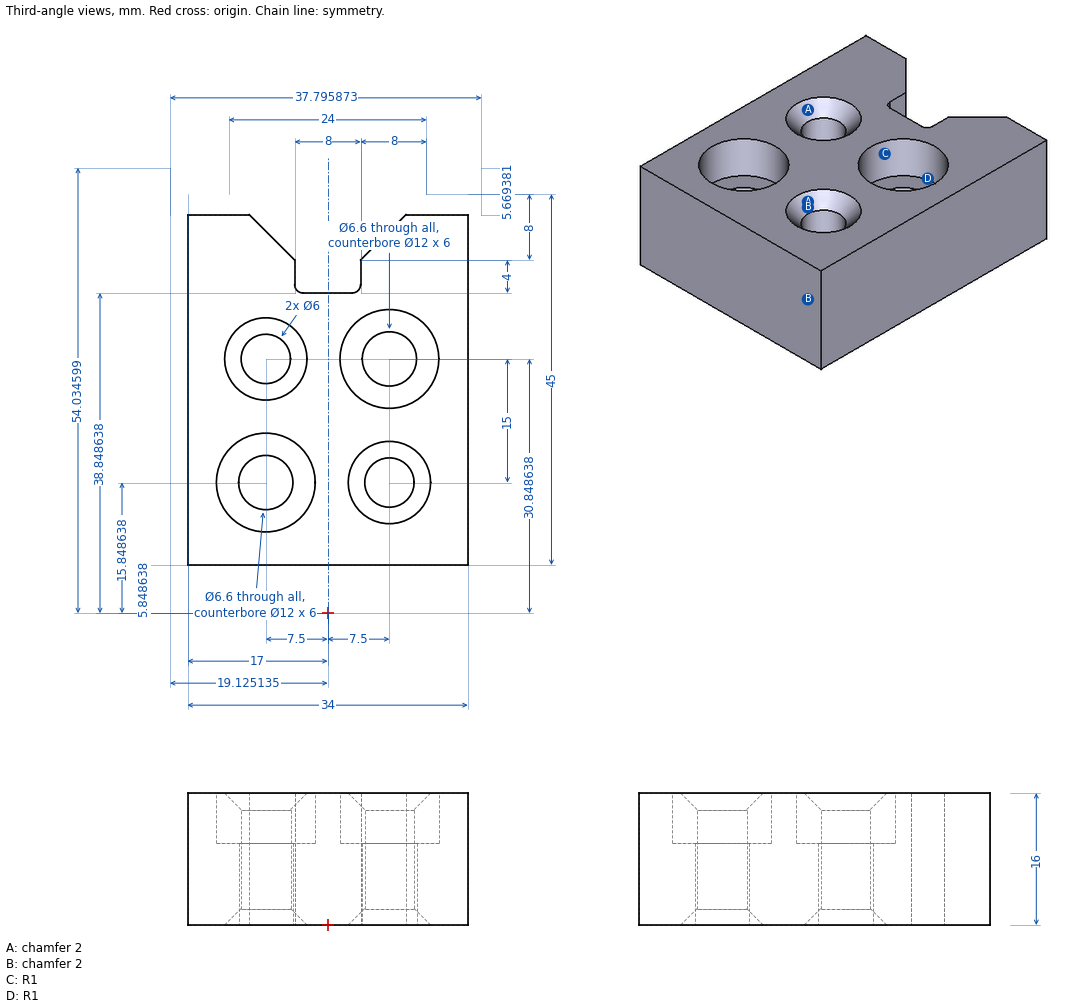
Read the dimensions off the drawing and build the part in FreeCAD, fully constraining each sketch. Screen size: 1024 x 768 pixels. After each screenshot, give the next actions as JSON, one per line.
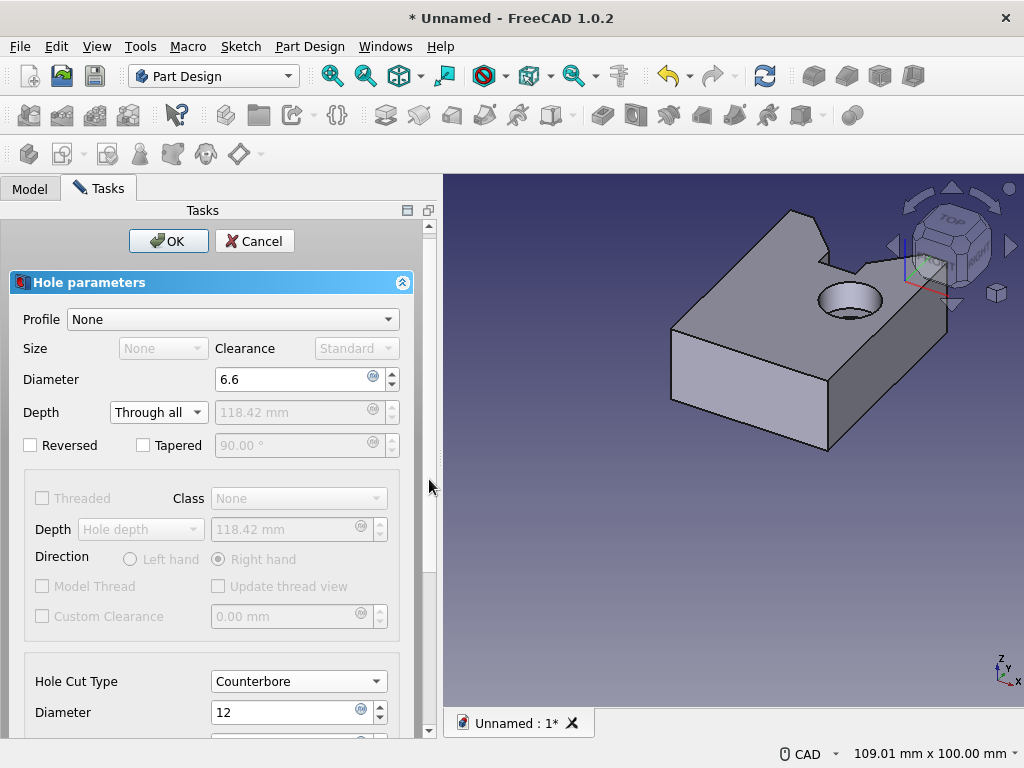
{"action": "left_click", "coordinate": [169, 249]}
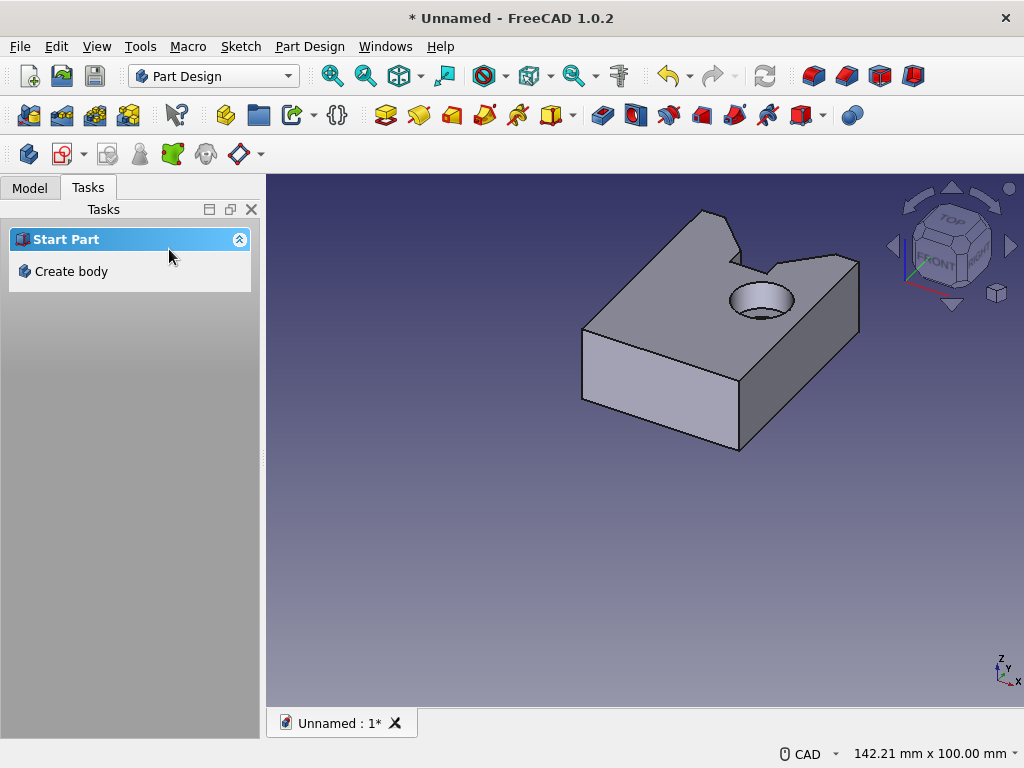
{"action": "left_click", "coordinate": [686, 329]}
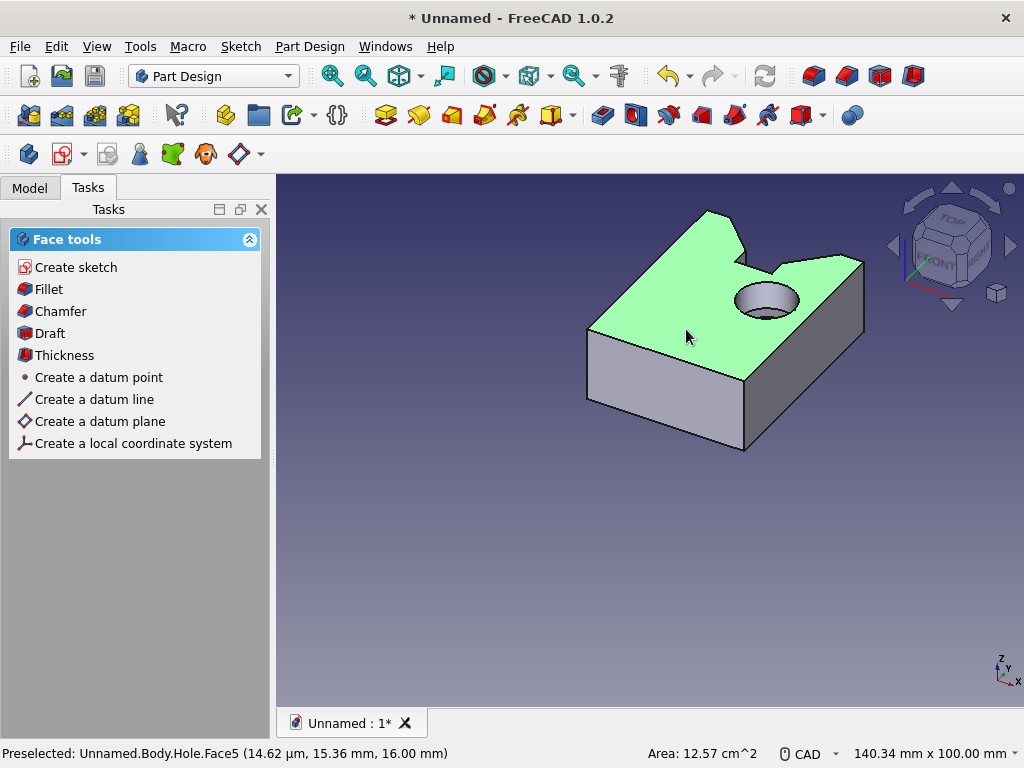
{"action": "left_click", "coordinate": [62, 154]}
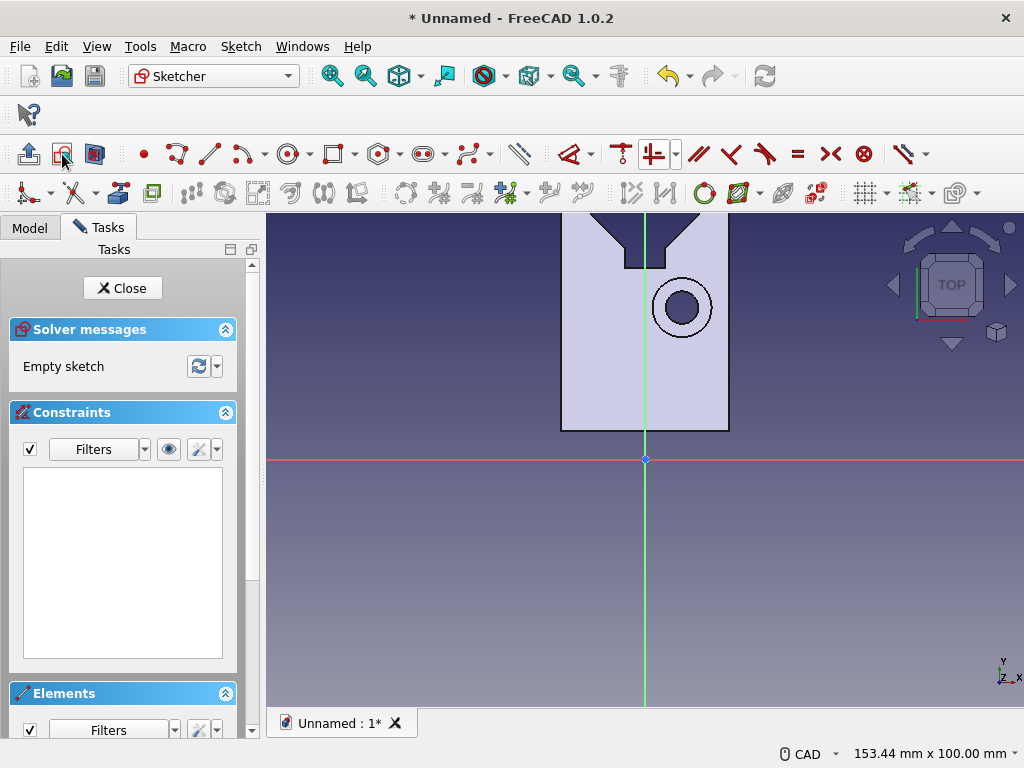
{"action": "scroll", "coordinate": [728, 275], "scroll_direction": "up", "scroll_amount": 3}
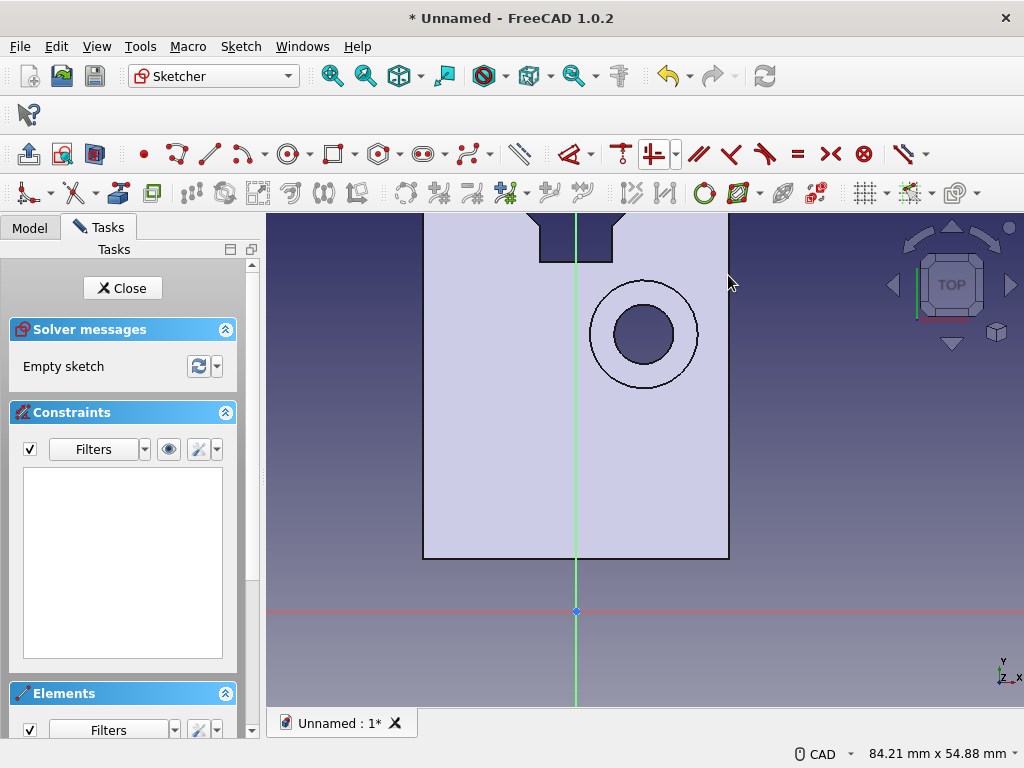
{"action": "left_click", "coordinate": [288, 154]}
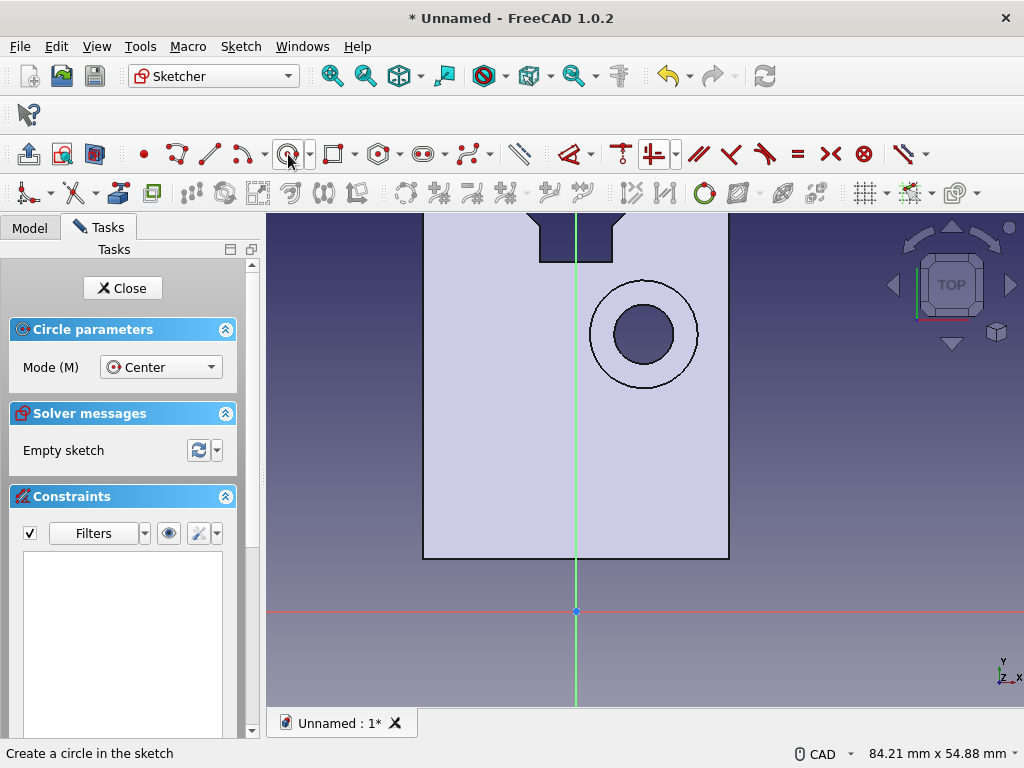
{"action": "left_click", "coordinate": [509, 334]}
{"action": "mouse_move", "coordinate": [528, 315]}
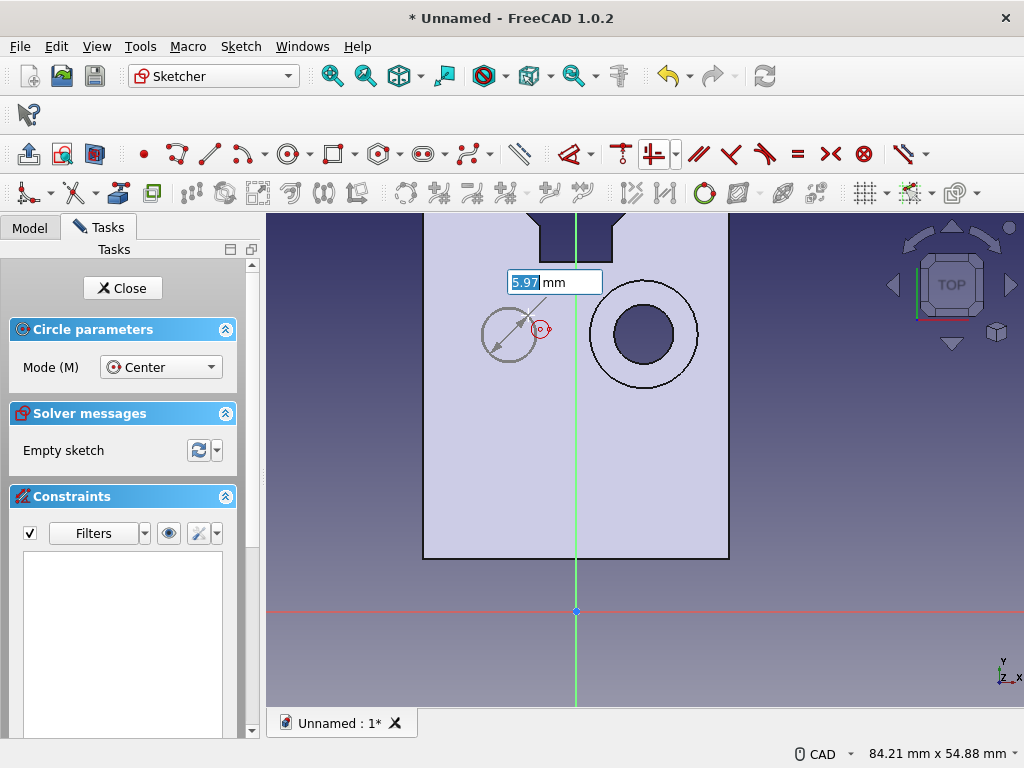
{"action": "type", "text": "6"}
{"action": "key", "text": "Return"}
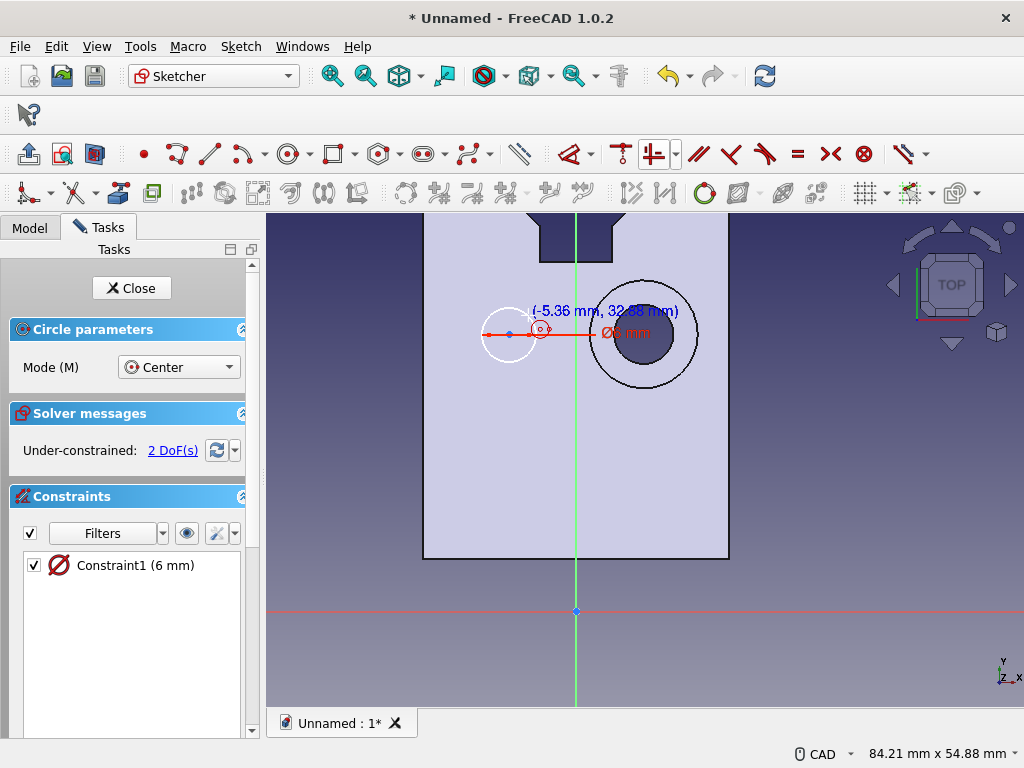
{"action": "left_click", "coordinate": [644, 469]}
{"action": "mouse_move", "coordinate": [663, 450]}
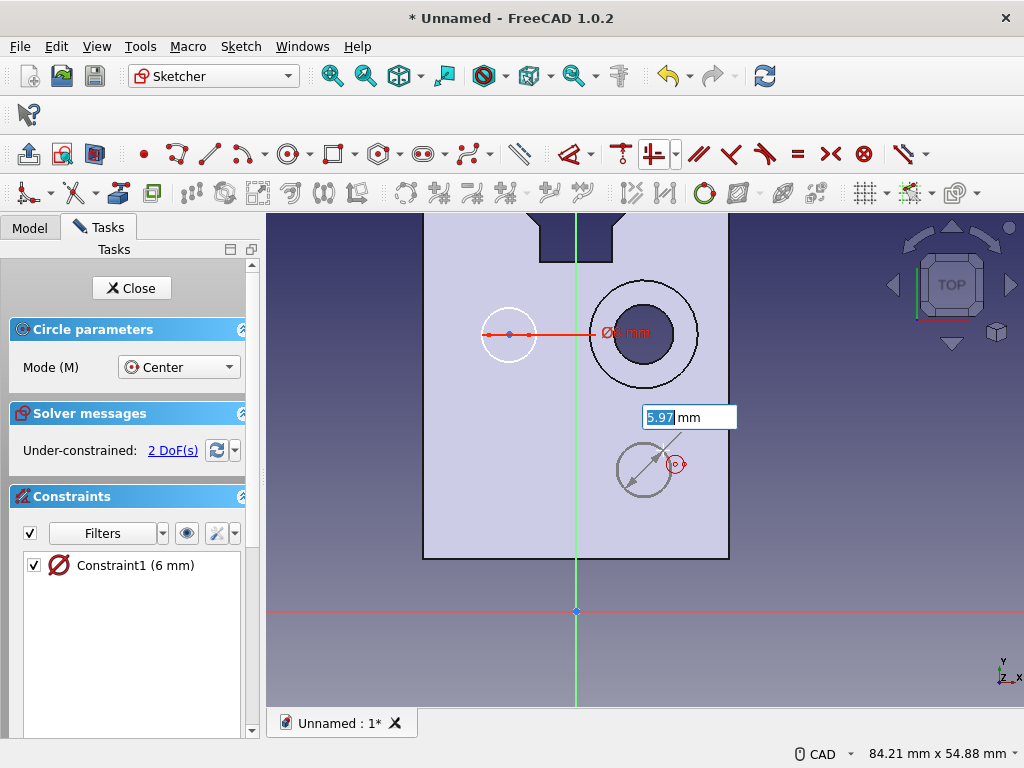
{"action": "type", "text": "6"}
{"action": "key", "text": "Return"}
{"action": "key", "text": "Escape"}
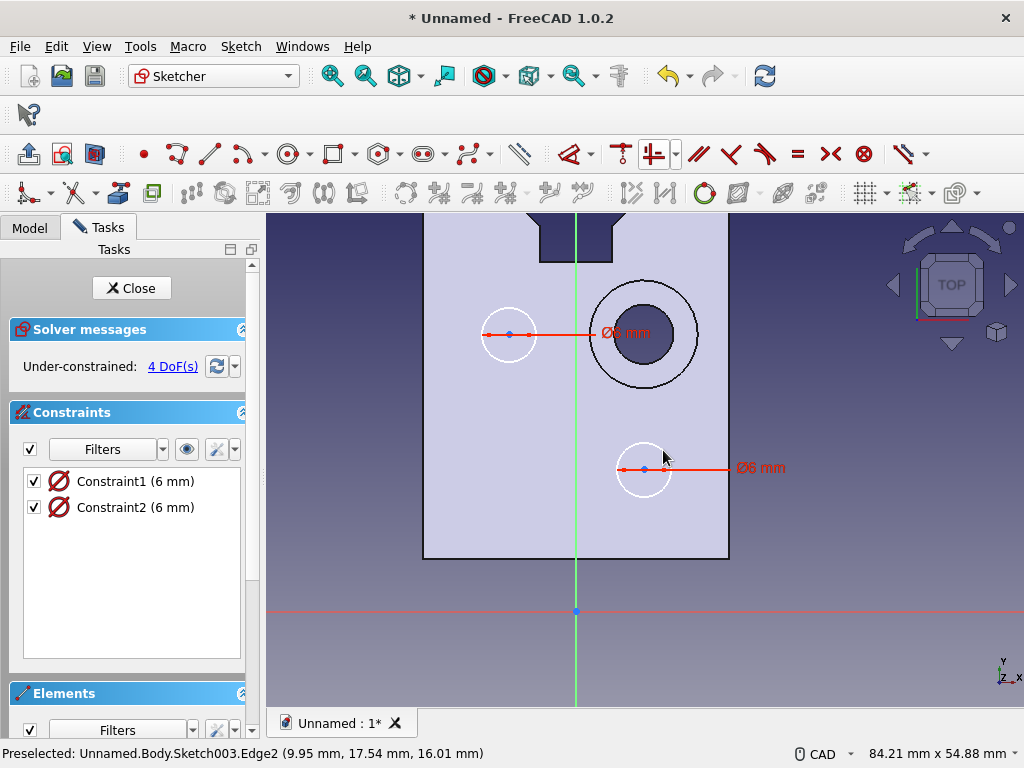
{"action": "left_click", "coordinate": [568, 154]}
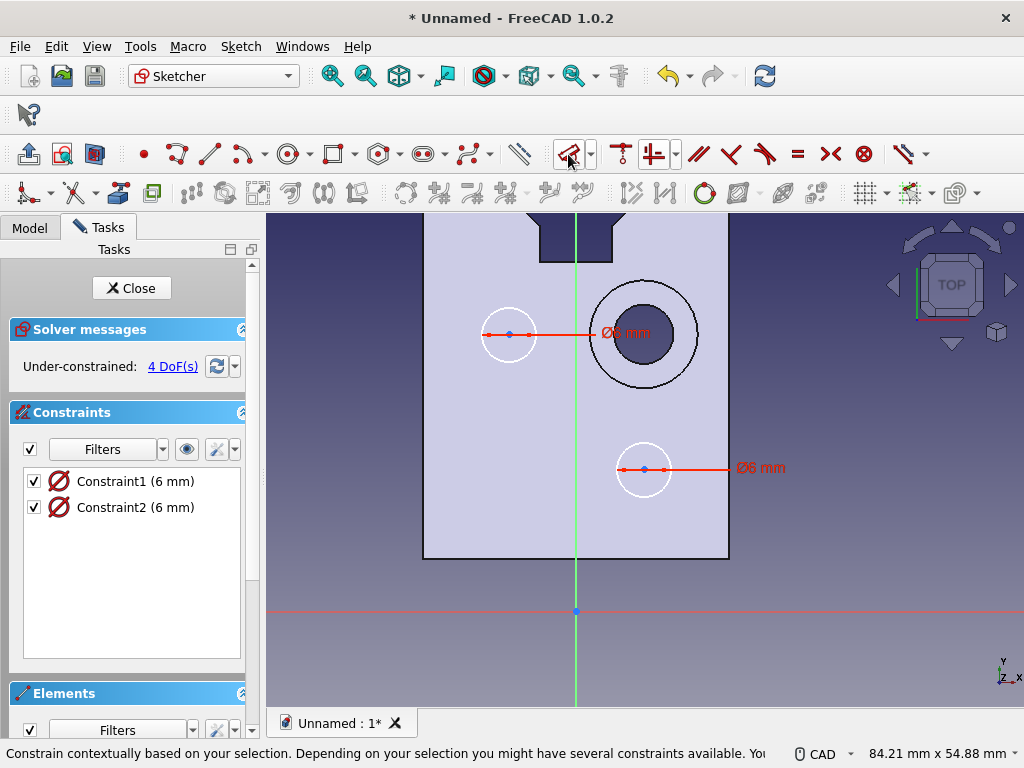
{"action": "left_click", "coordinate": [509, 335]}
{"action": "left_click", "coordinate": [543, 646]}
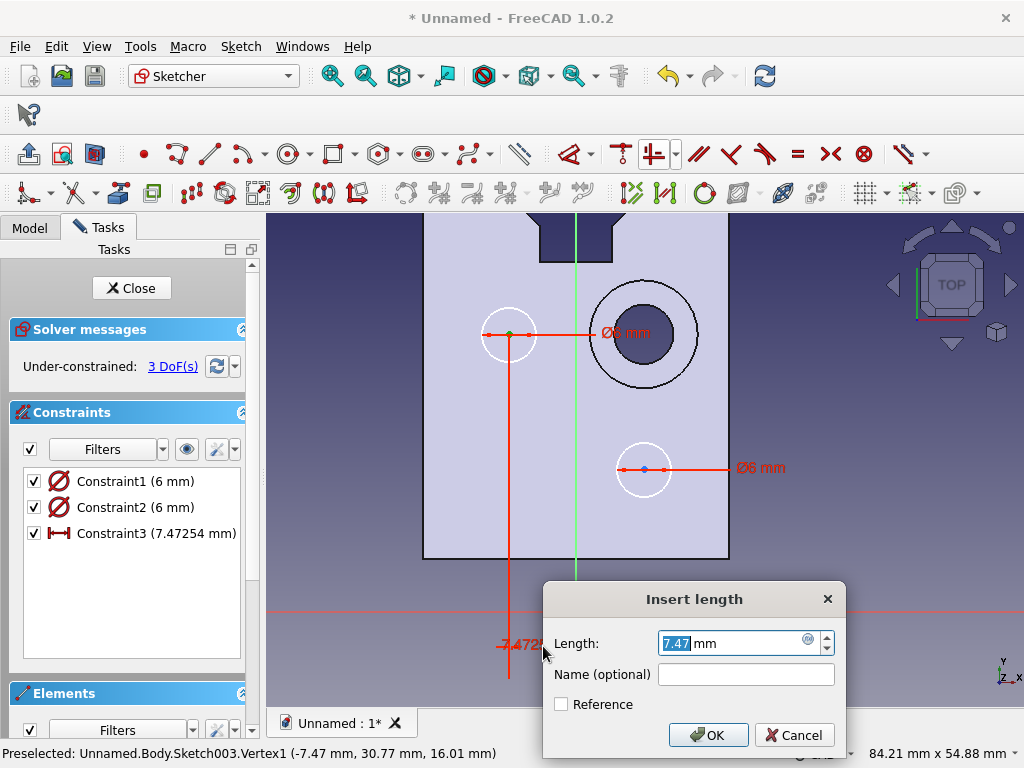
{"action": "type", "text": "7.5"}
{"action": "key", "text": "Return"}